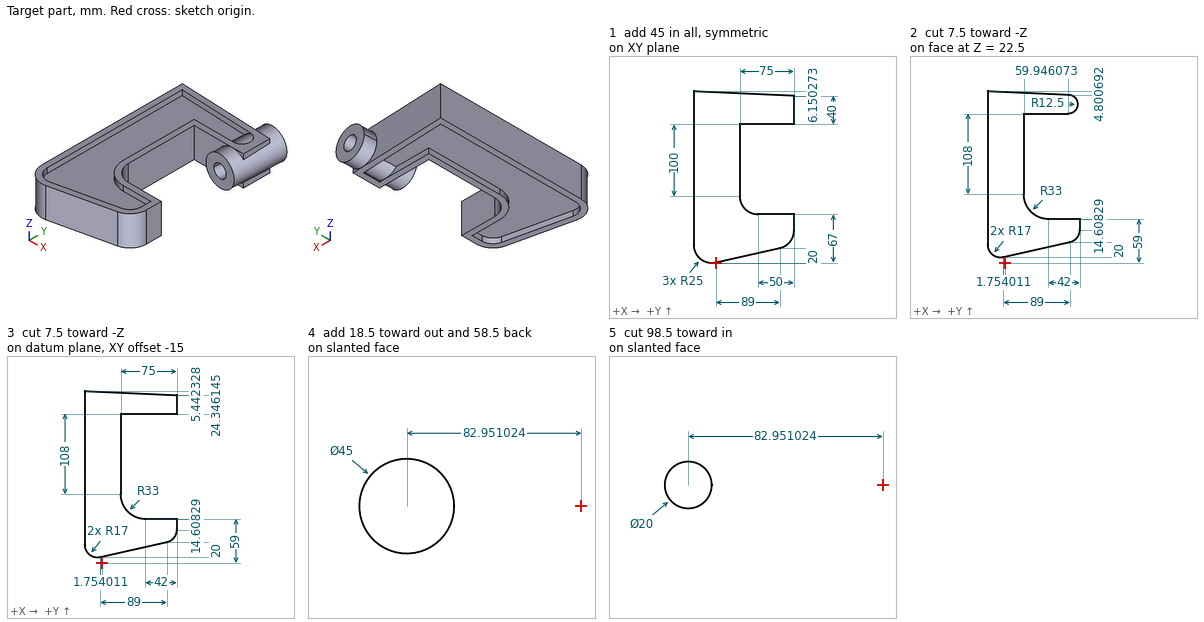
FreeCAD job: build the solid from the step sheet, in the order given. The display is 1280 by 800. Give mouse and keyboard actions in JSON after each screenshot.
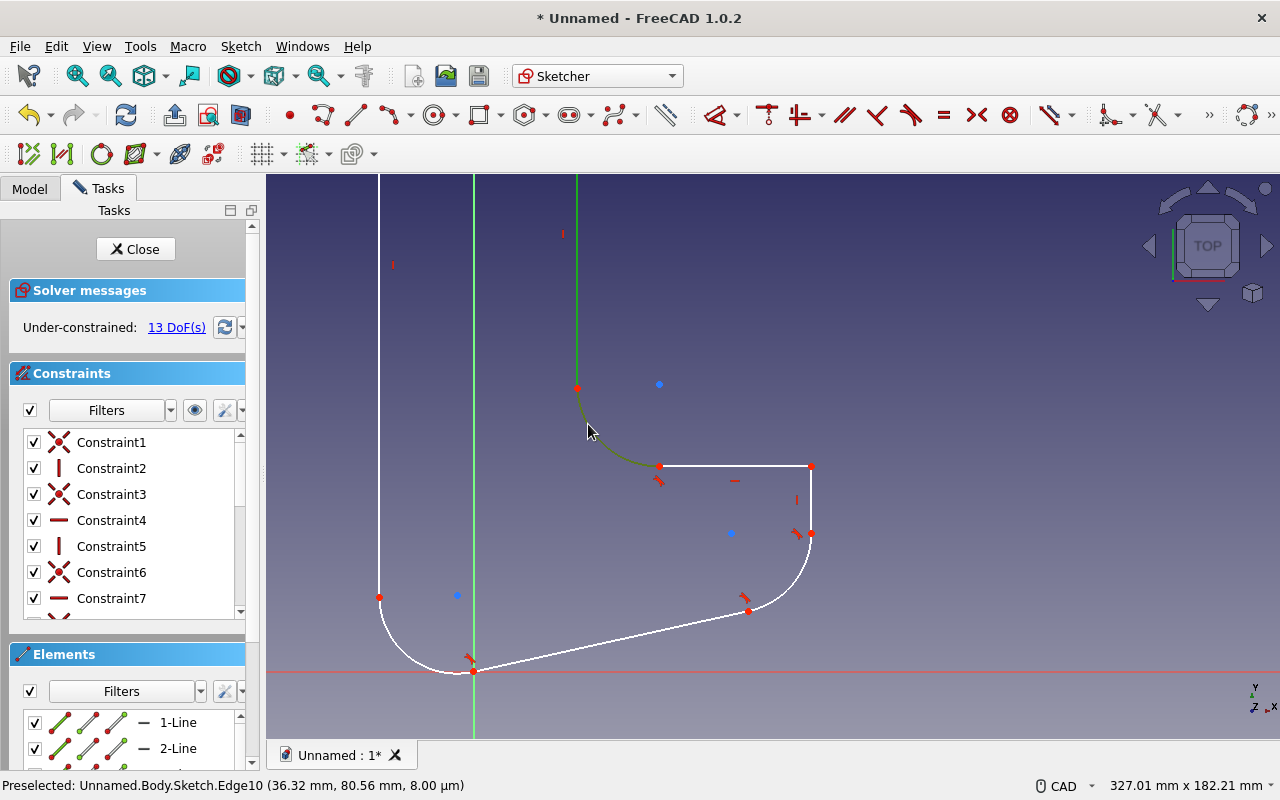
{"action": "key", "text": "t"}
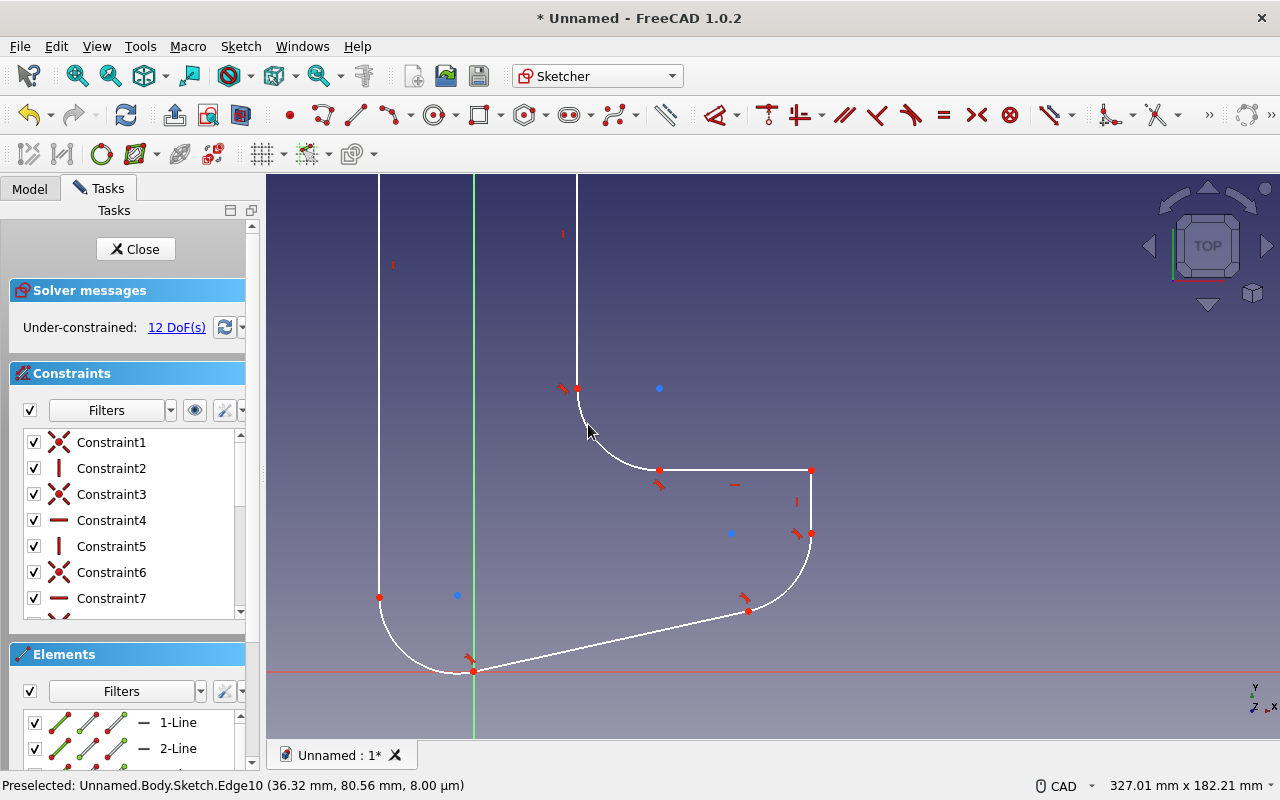
{"action": "left_click", "coordinate": [379, 398]}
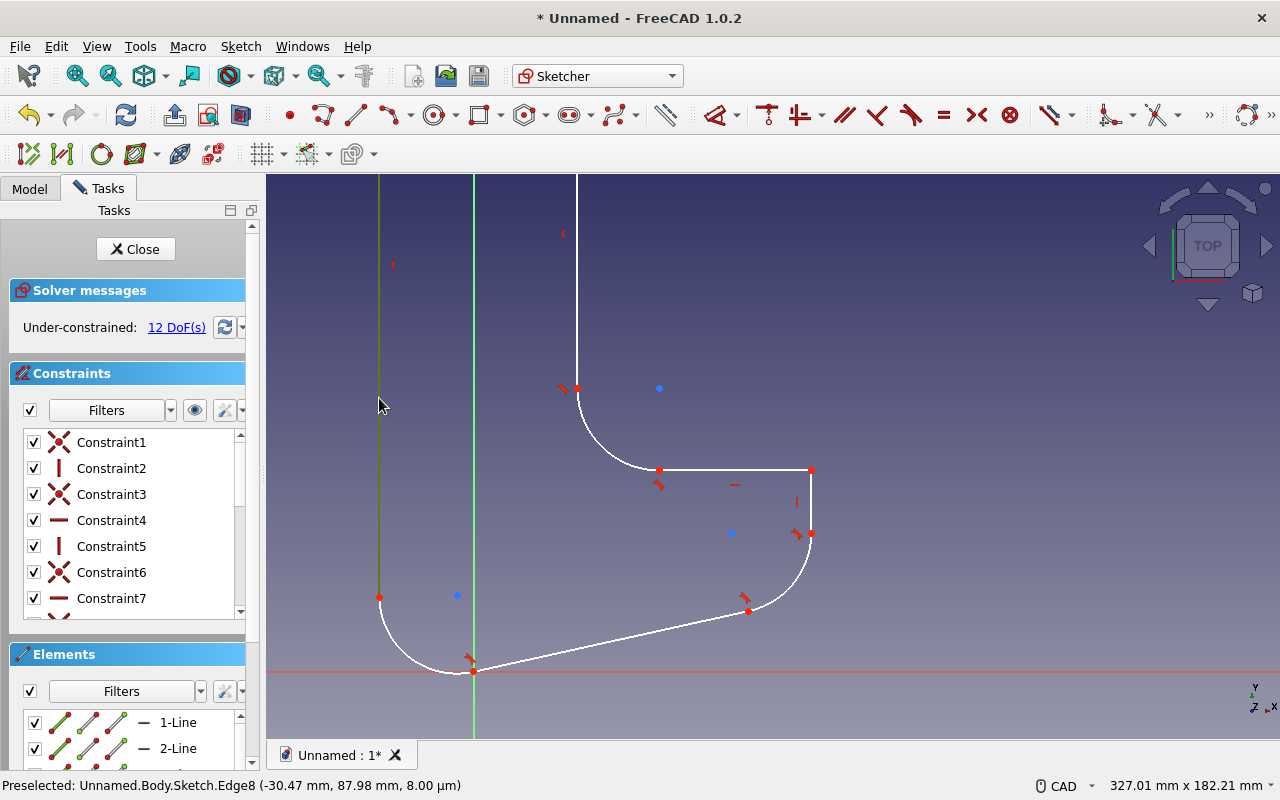
{"action": "left_click", "coordinate": [391, 637]}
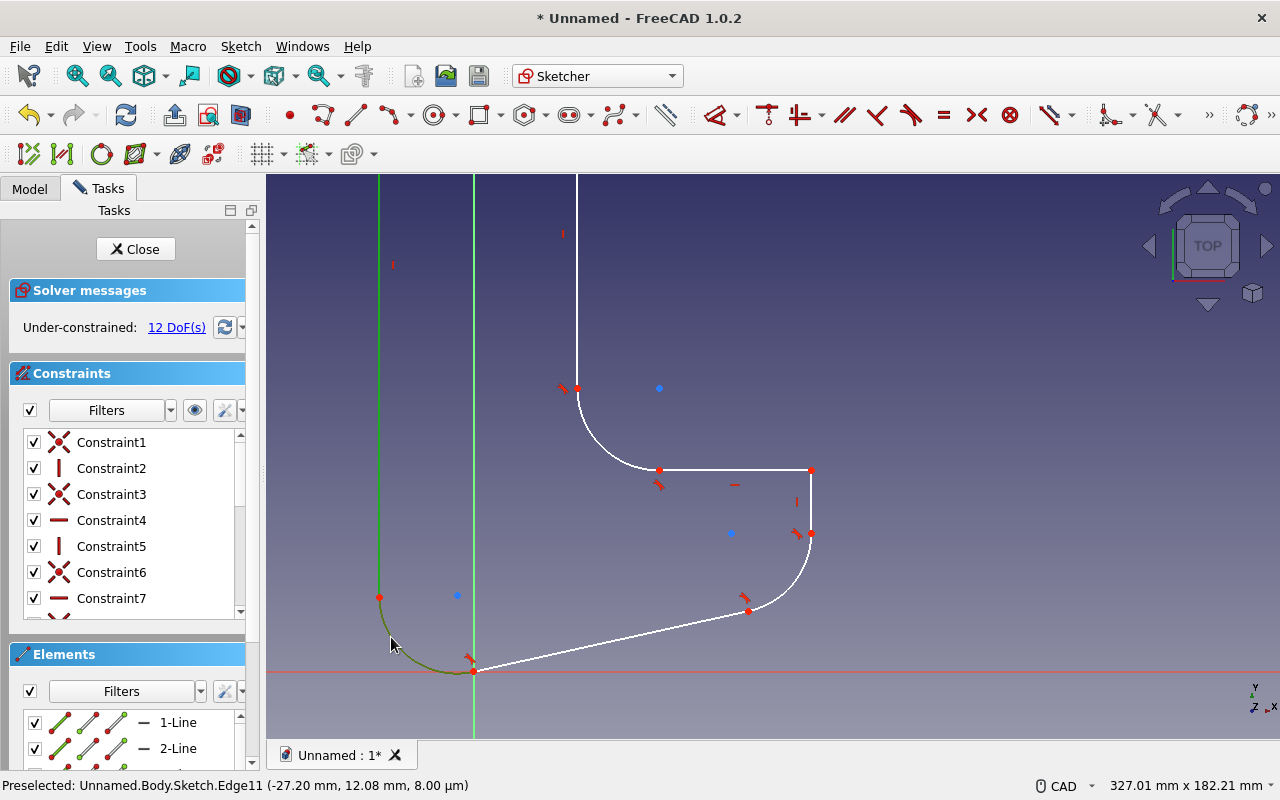
{"action": "left_click", "coordinate": [911, 116]}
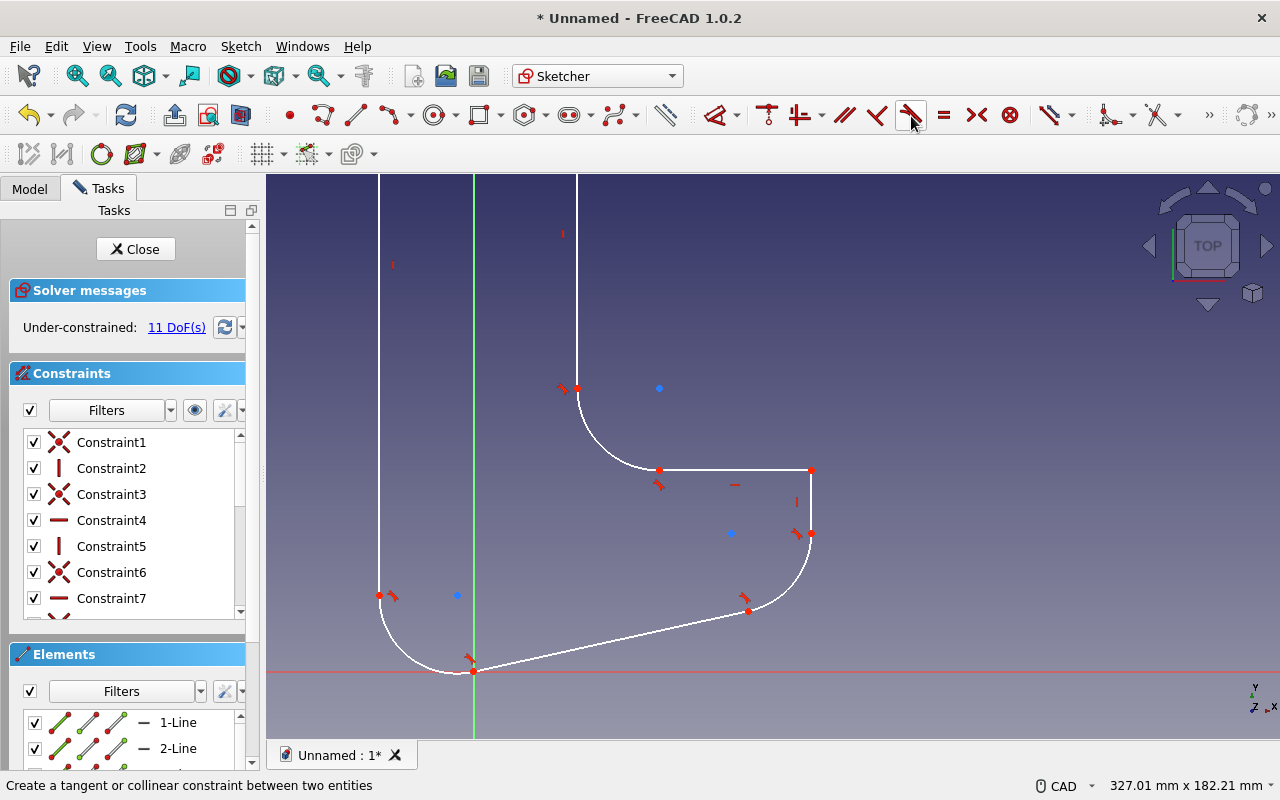
{"action": "left_click", "coordinate": [778, 598]}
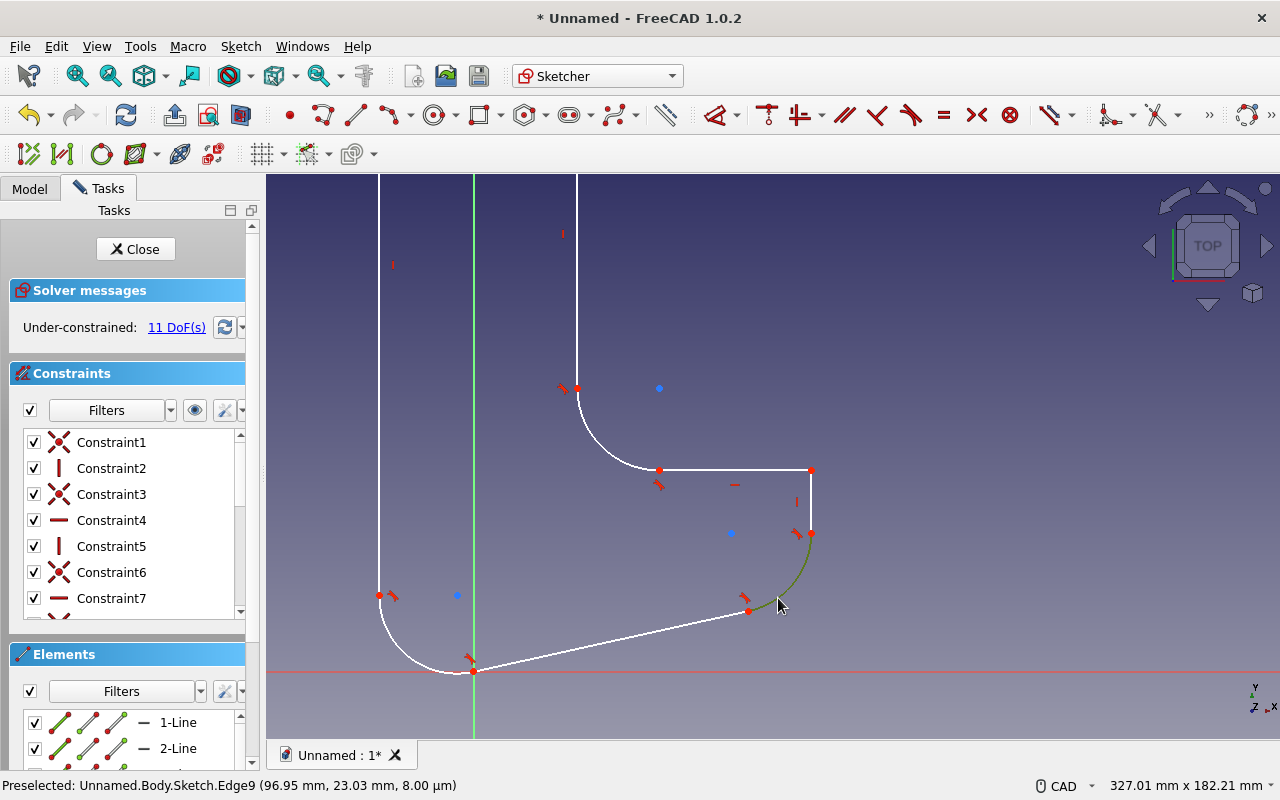
{"action": "left_click", "coordinate": [586, 426]}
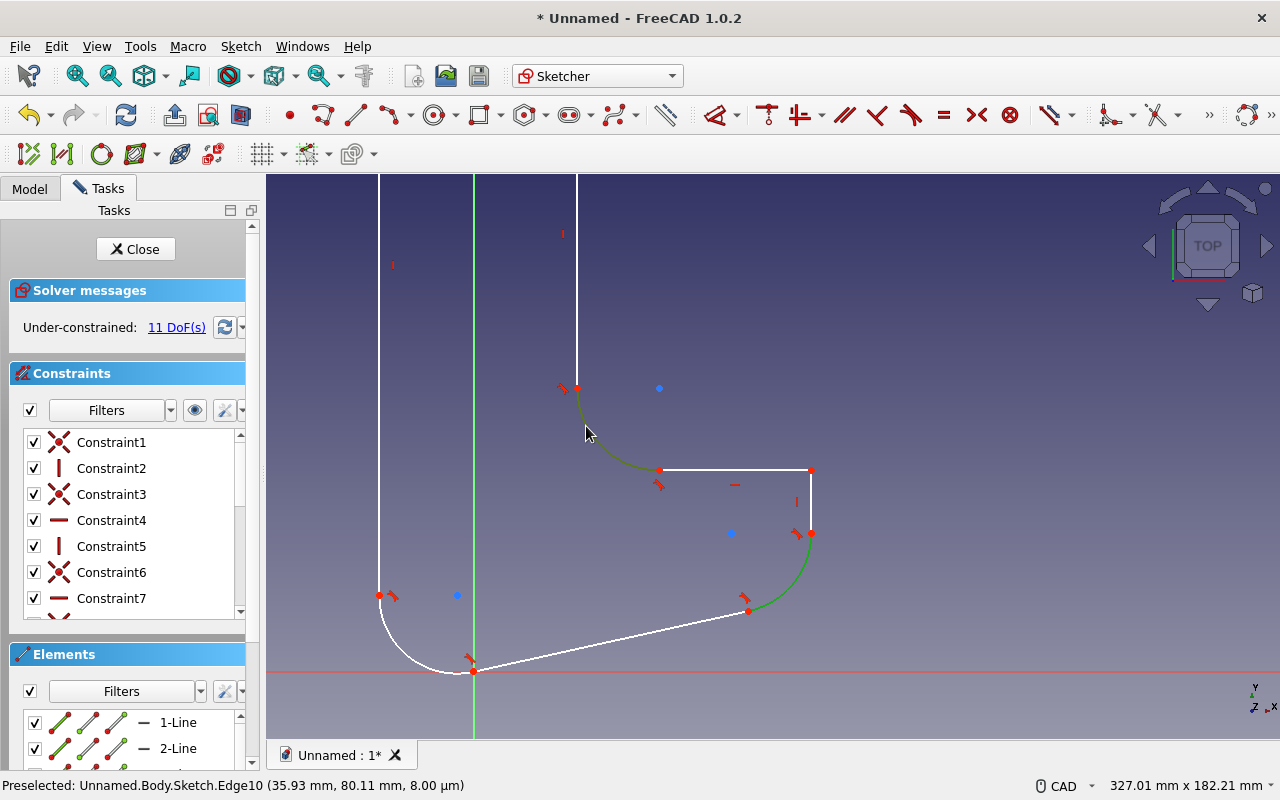
{"action": "left_click", "coordinate": [390, 636]}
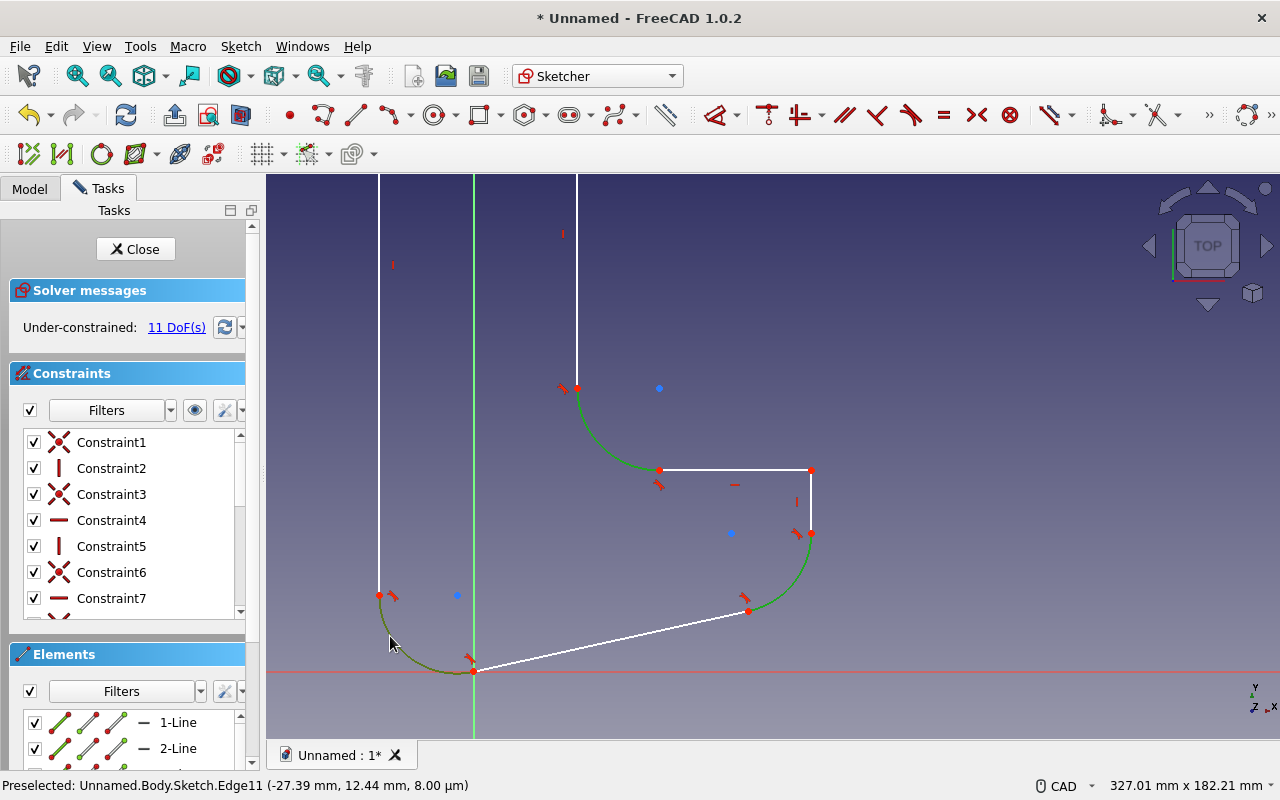
{"action": "left_click", "coordinate": [944, 116]}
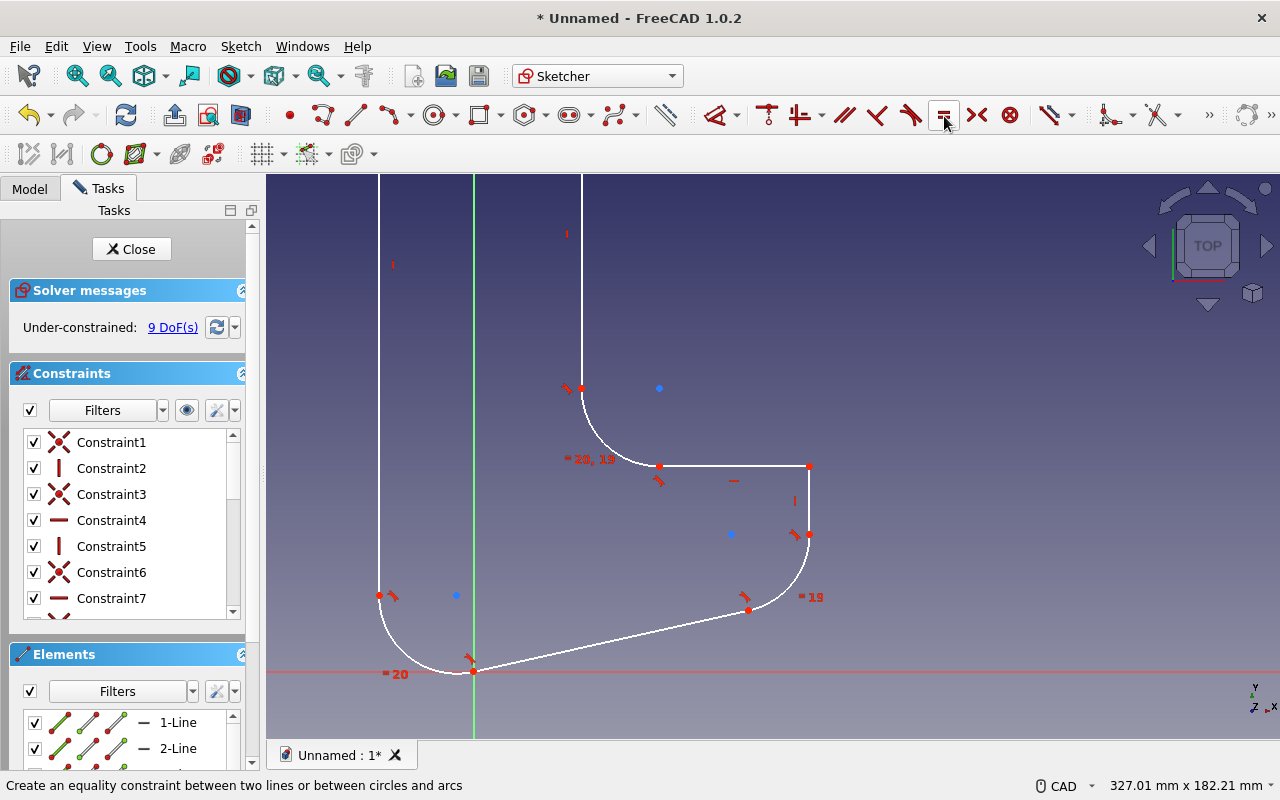
{"action": "left_click", "coordinate": [714, 116]}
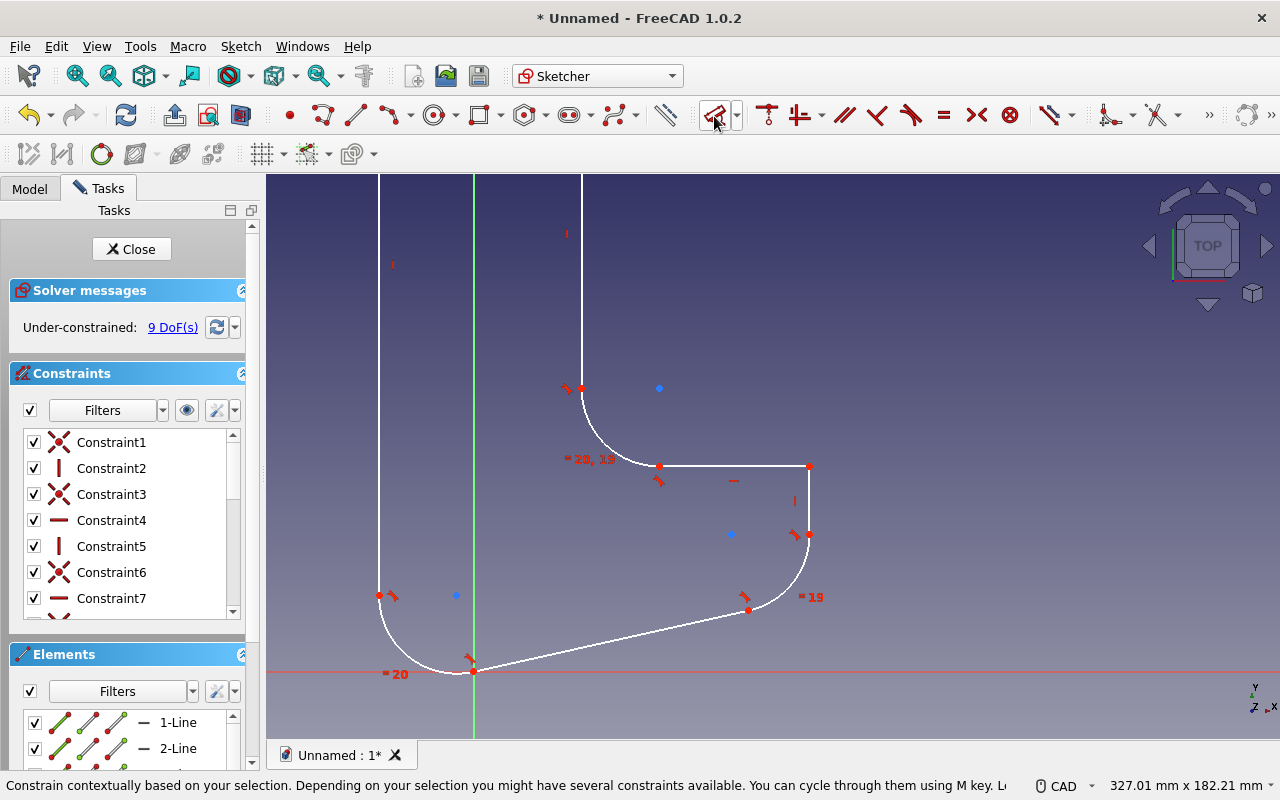
{"action": "left_click", "coordinate": [777, 598]}
{"action": "left_click", "coordinate": [796, 624]}